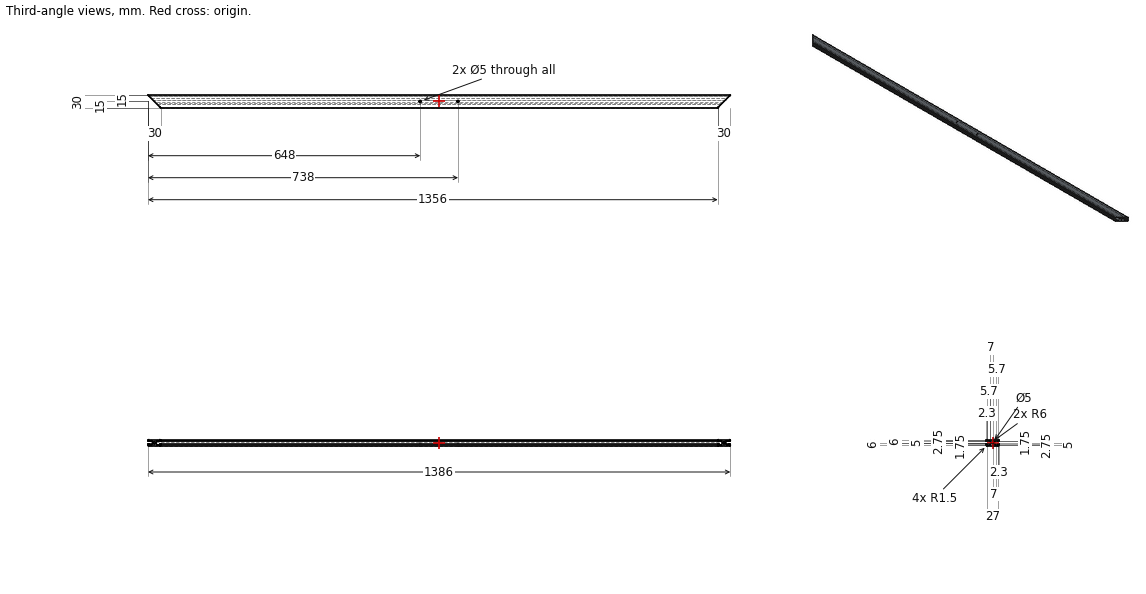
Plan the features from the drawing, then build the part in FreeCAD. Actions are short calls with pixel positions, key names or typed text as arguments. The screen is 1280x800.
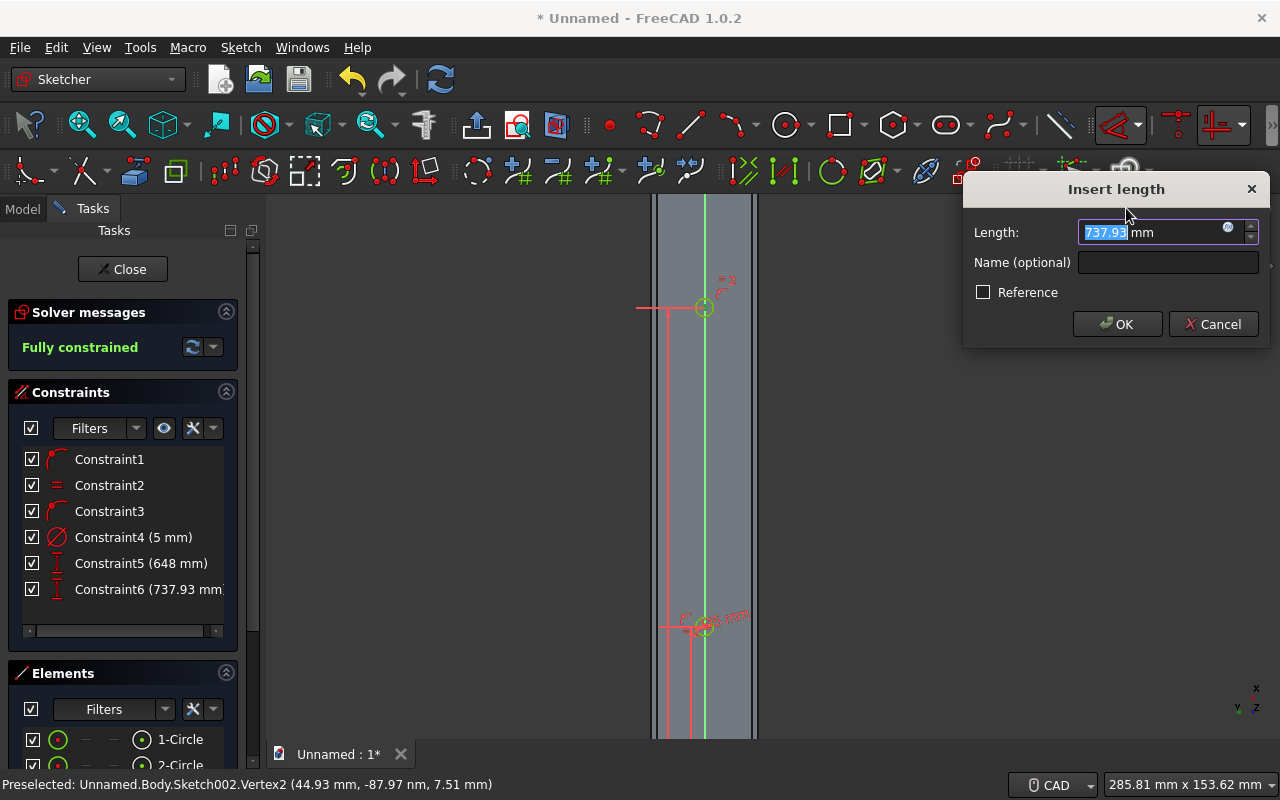
text(738)
key(Return)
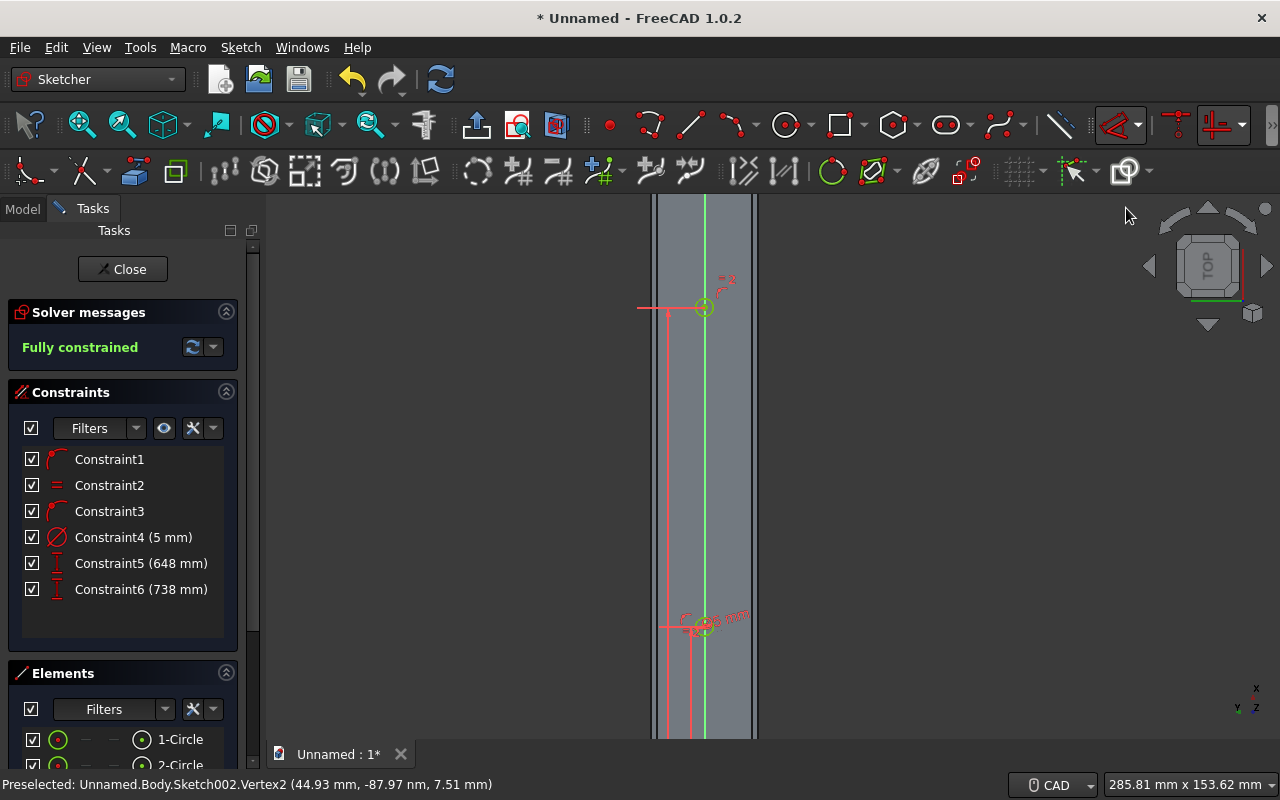
click(123, 269)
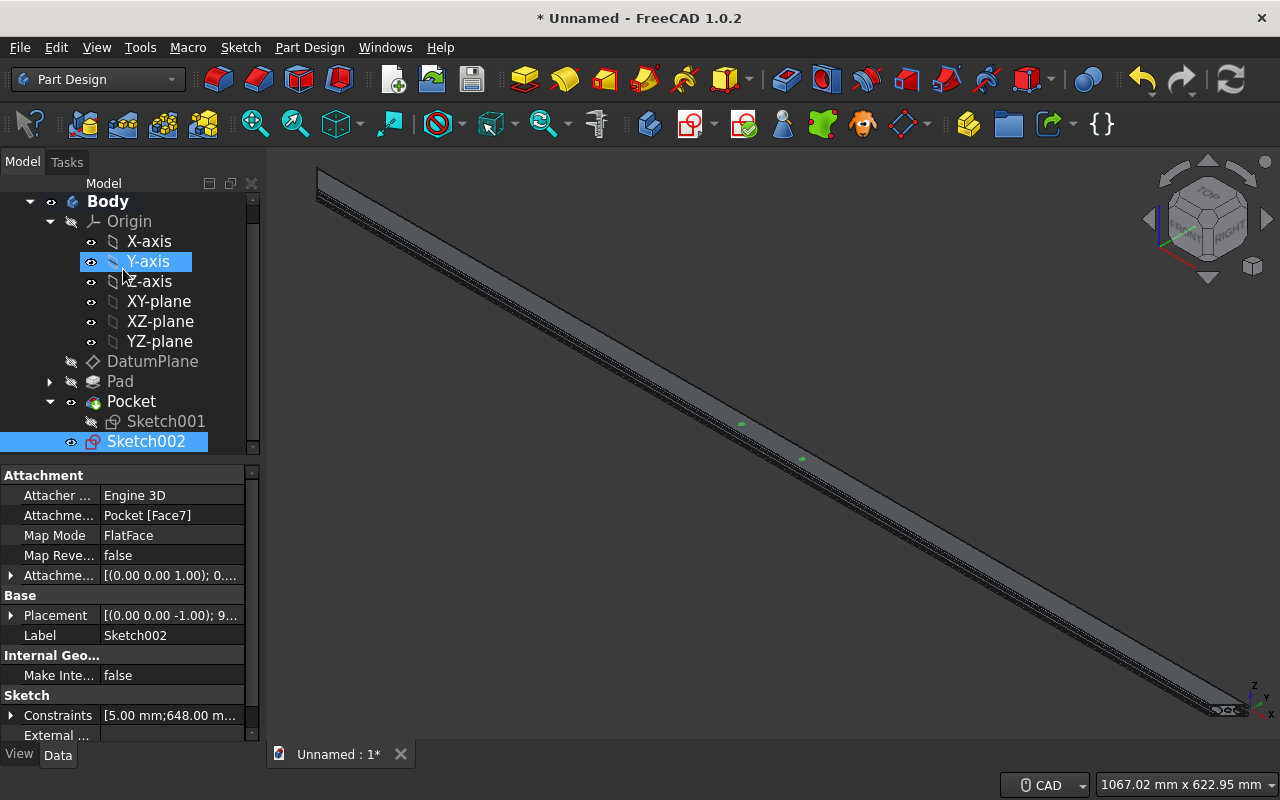
click(828, 80)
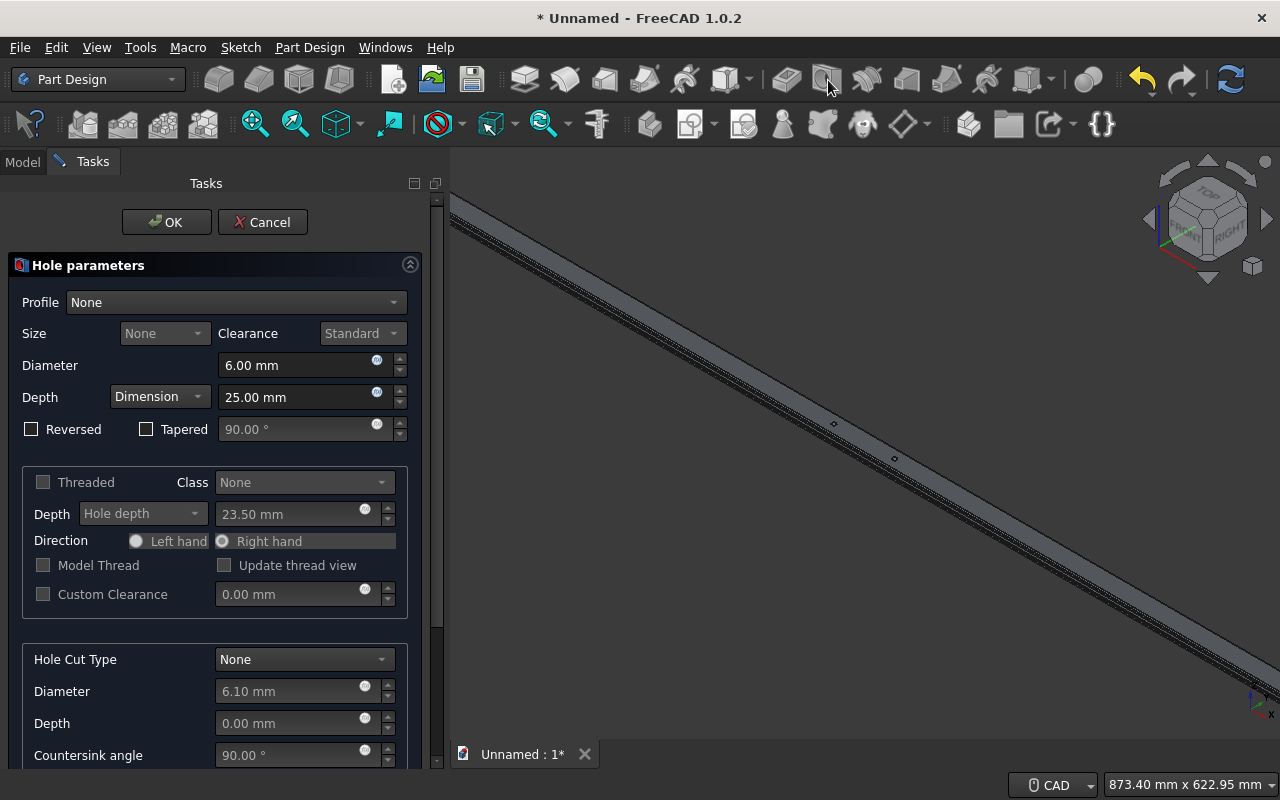
triple_click(305, 365)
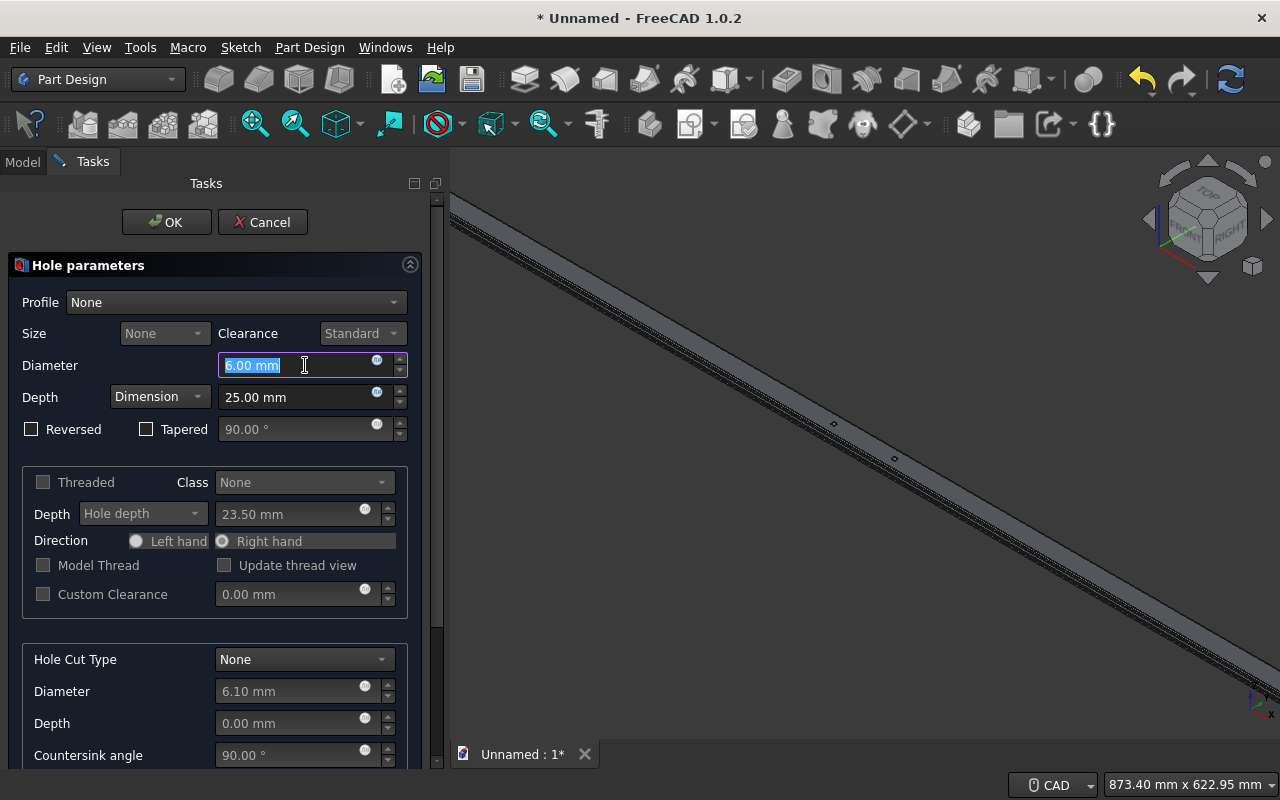
text(5)
key(Tab)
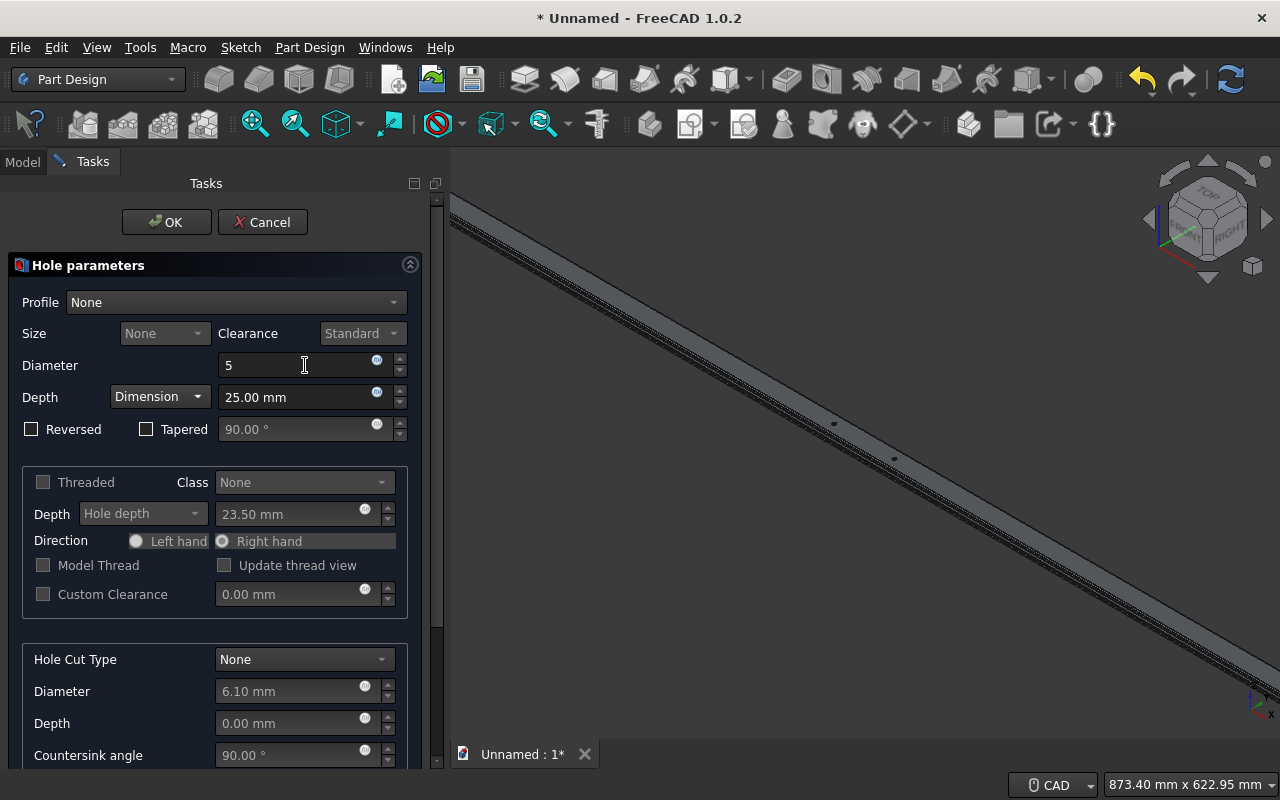
click(161, 396)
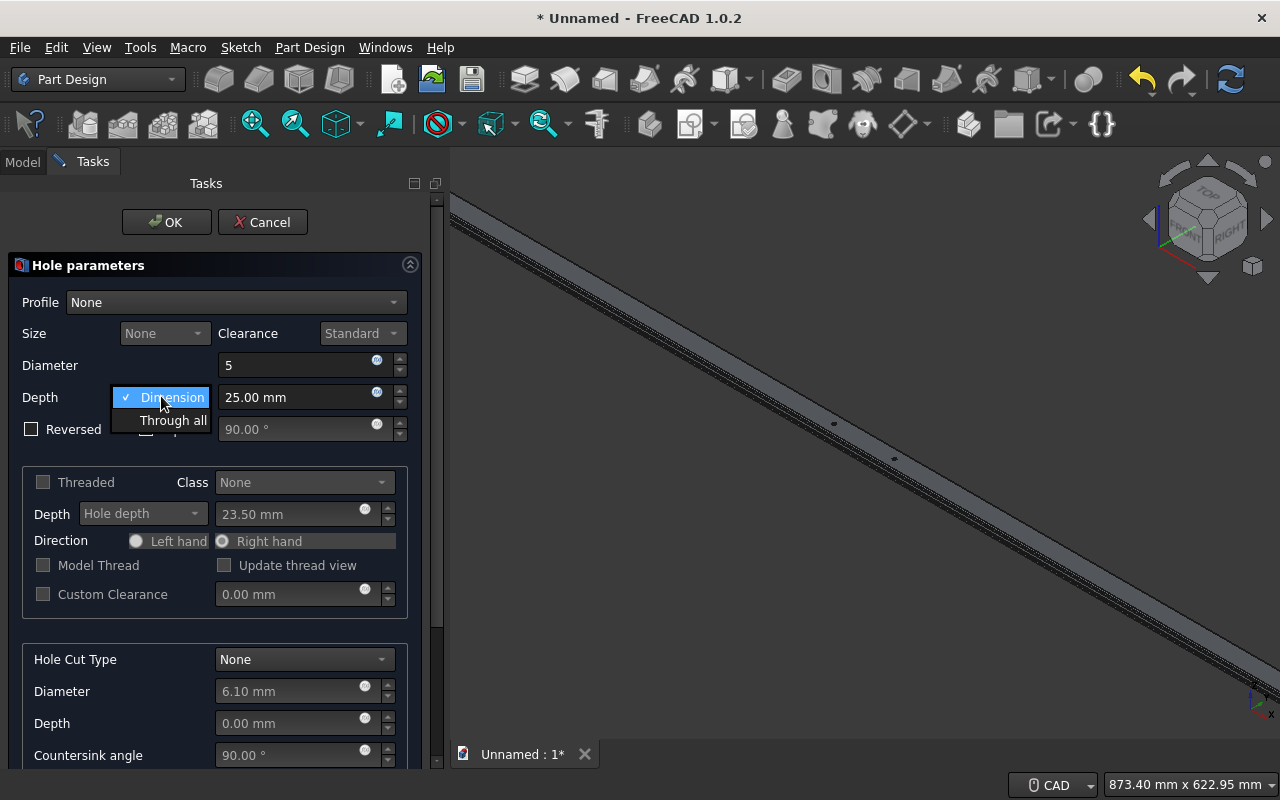
click(160, 420)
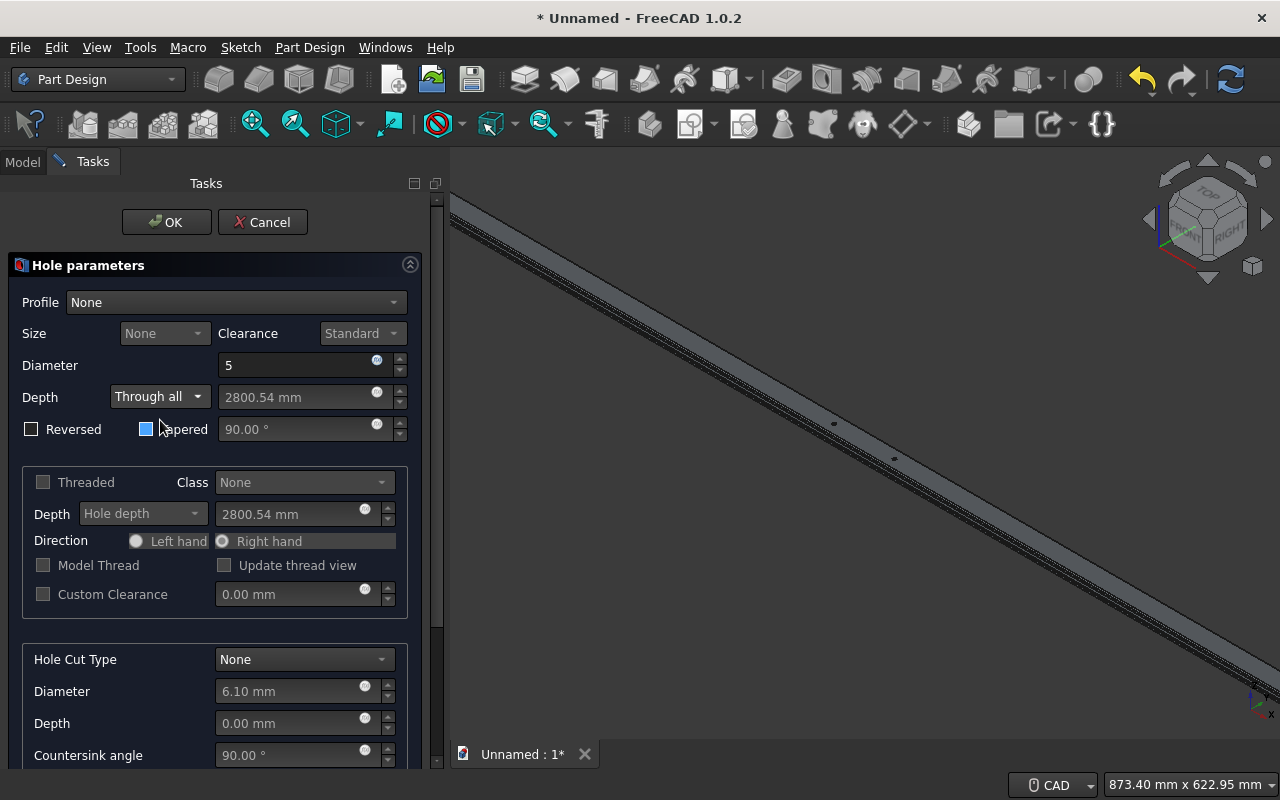
click(167, 222)